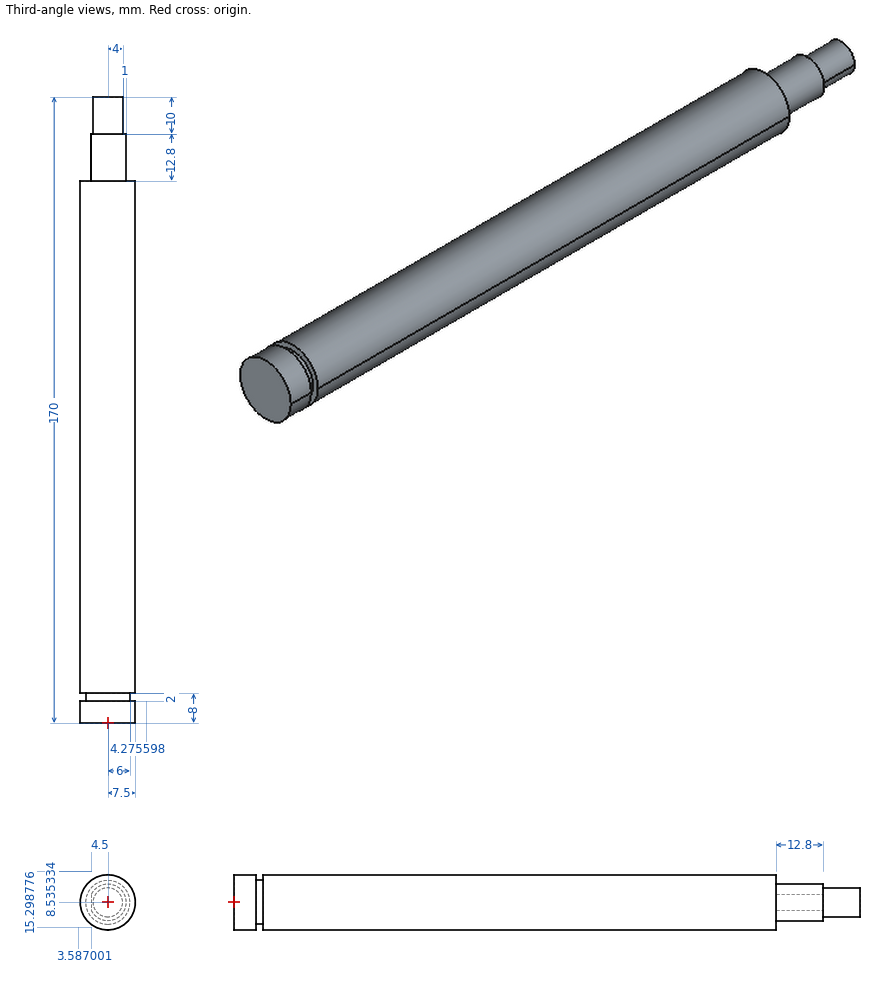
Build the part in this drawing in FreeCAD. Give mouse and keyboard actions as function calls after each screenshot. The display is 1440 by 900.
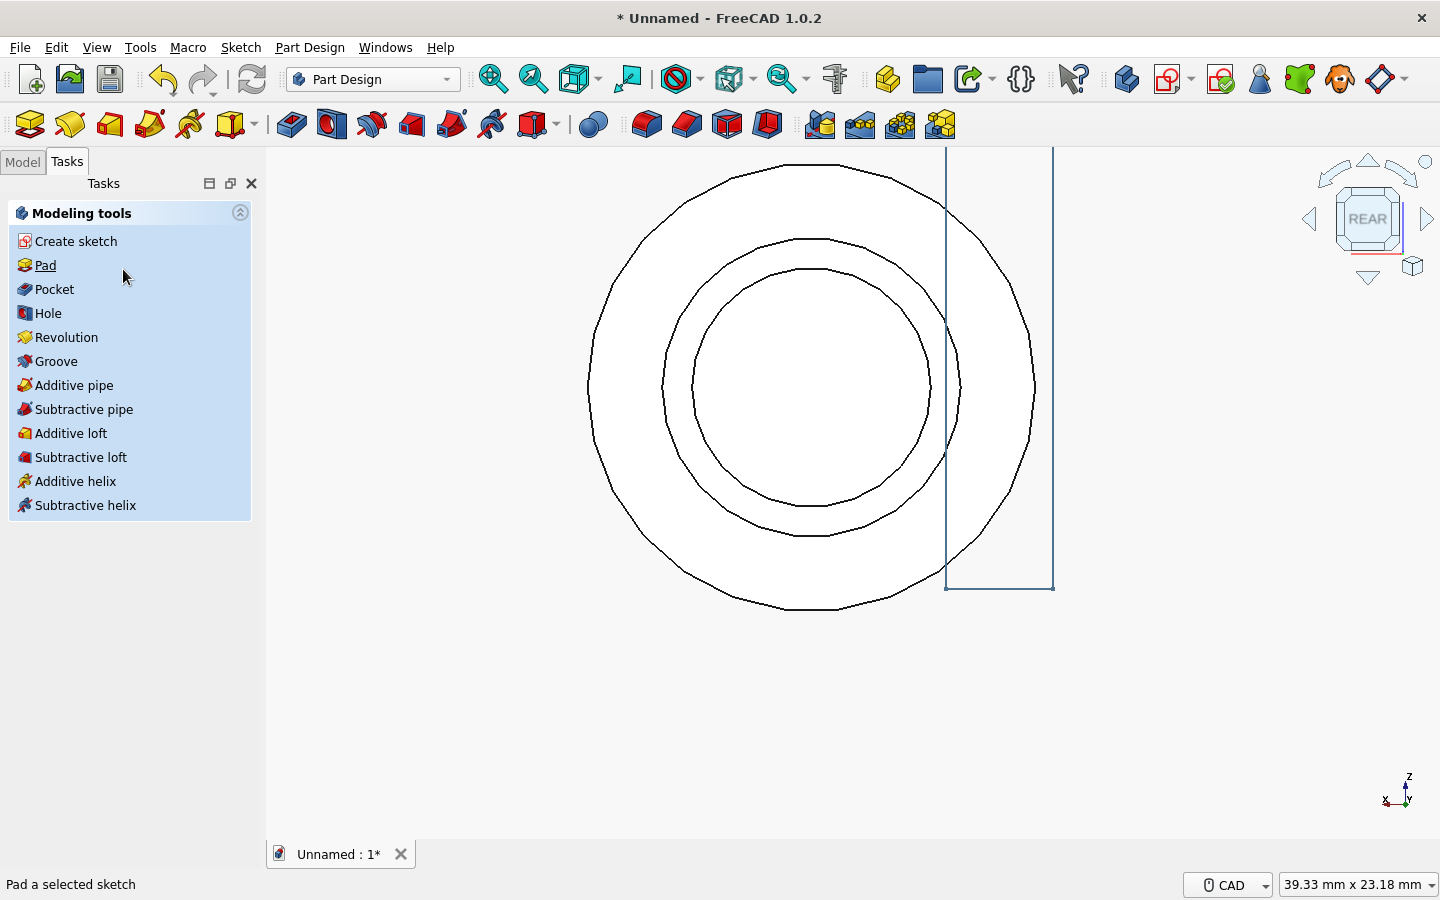
click(292, 124)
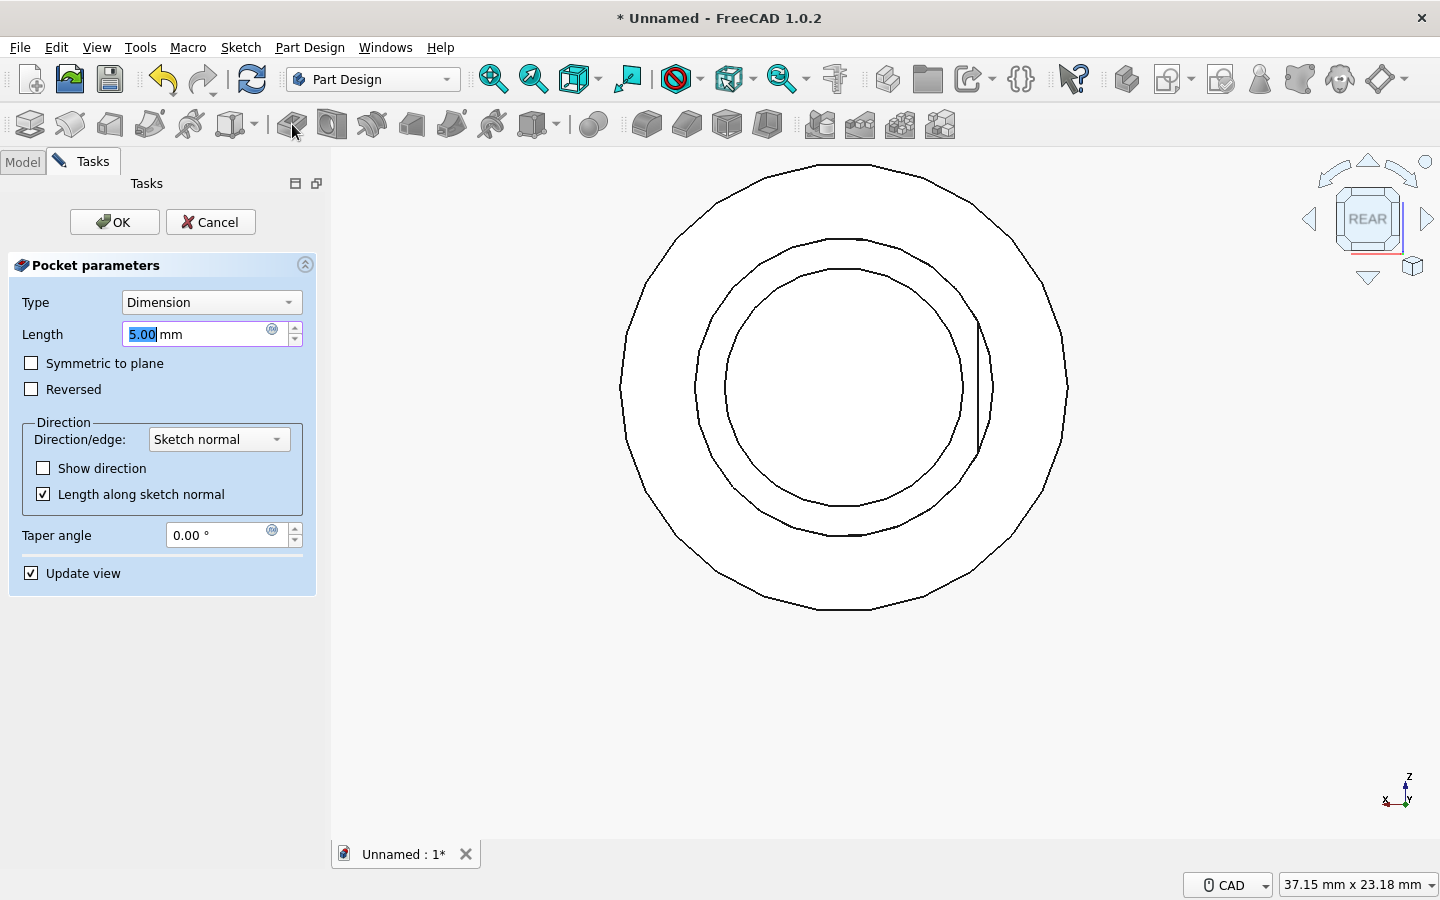
text(12.8)
key(Tab)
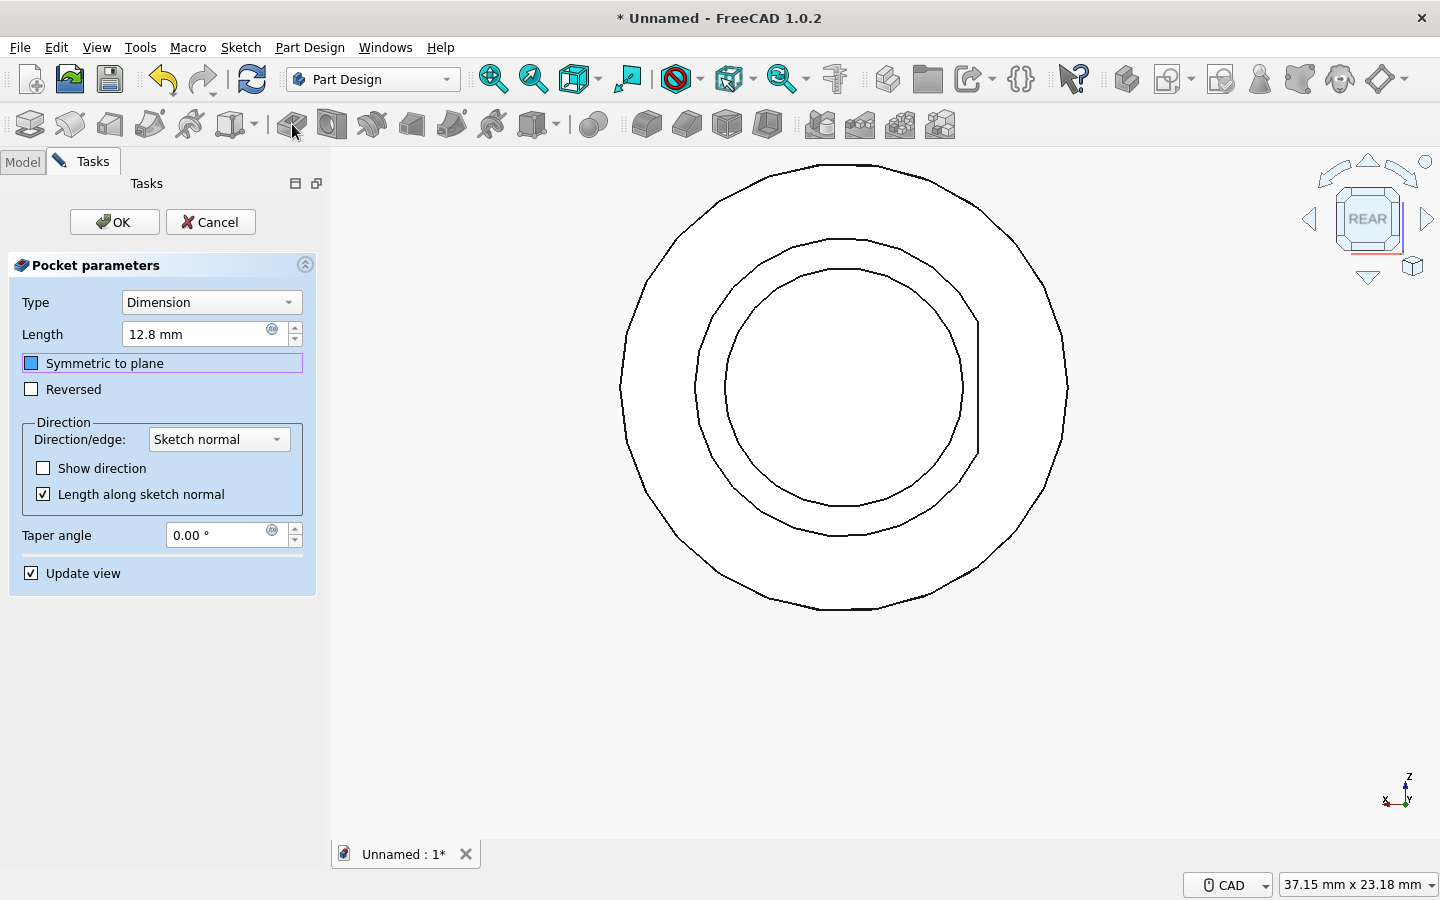
click(115, 222)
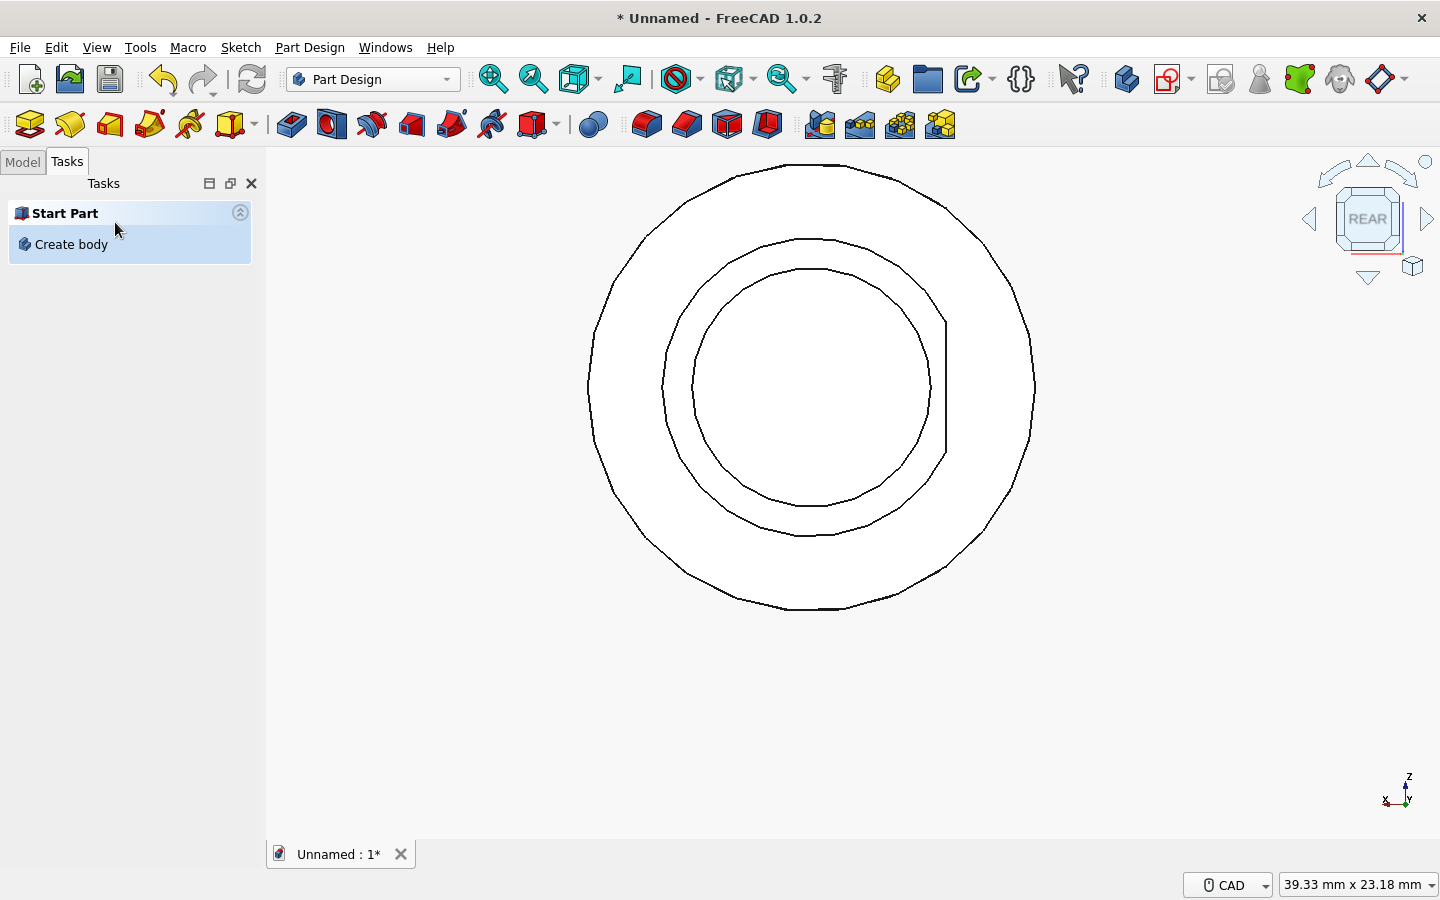
click(1168, 80)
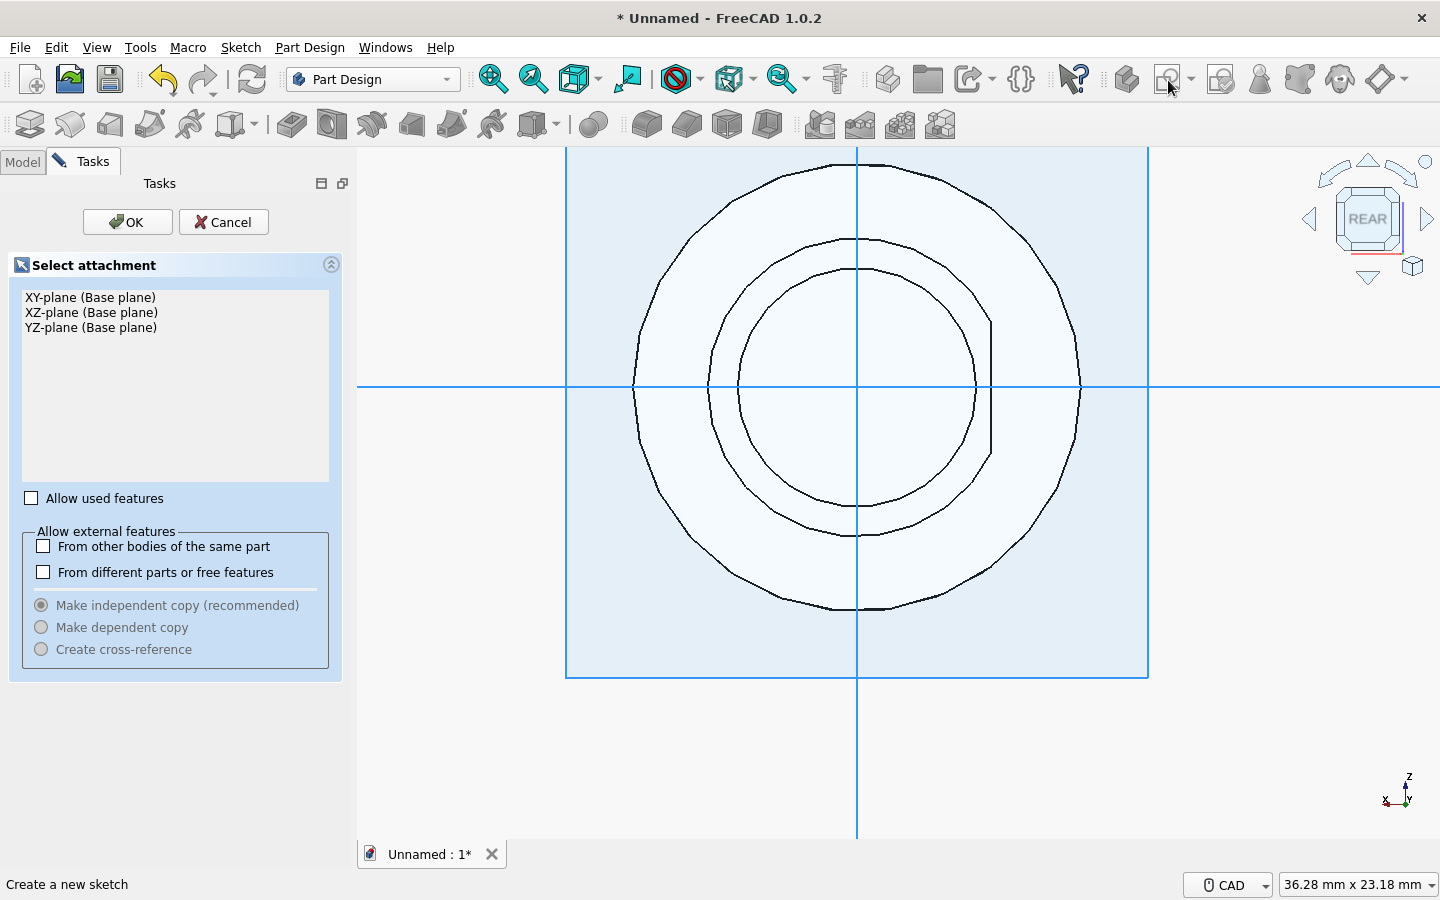
click(82, 298)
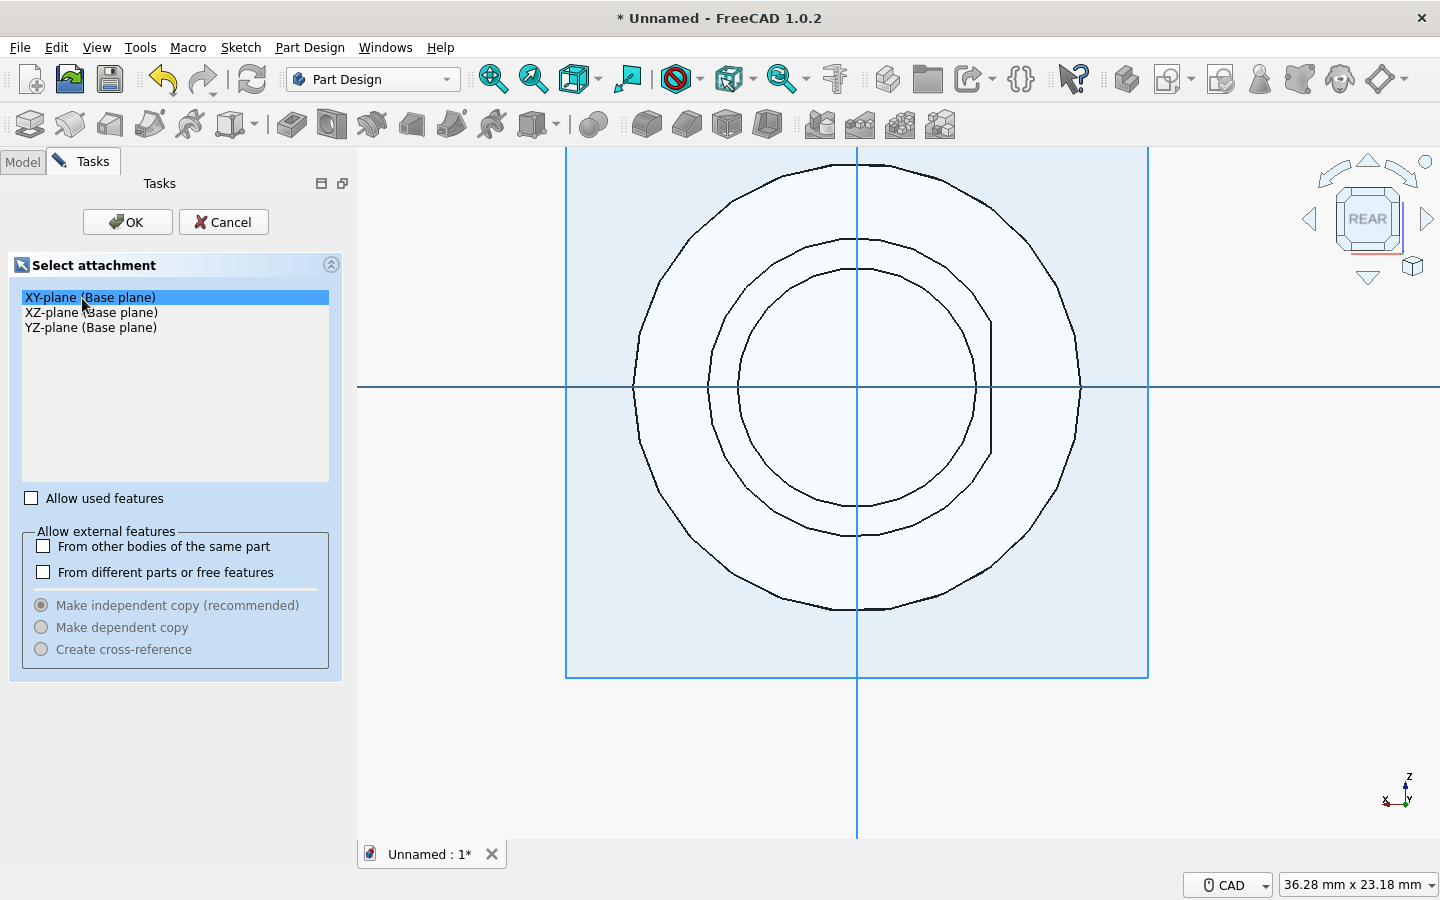
click(128, 222)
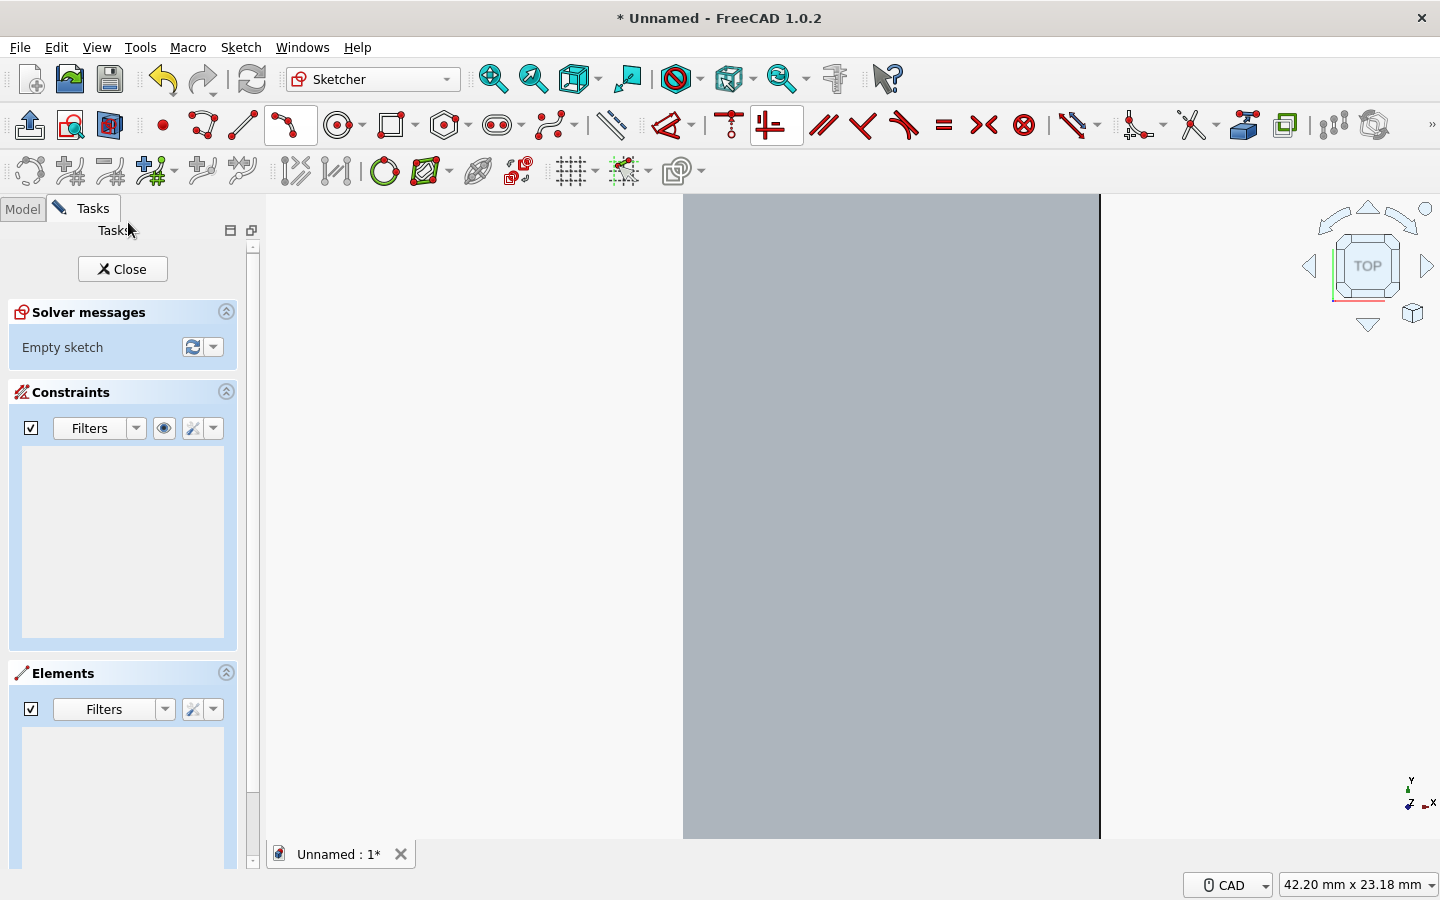
click(110, 126)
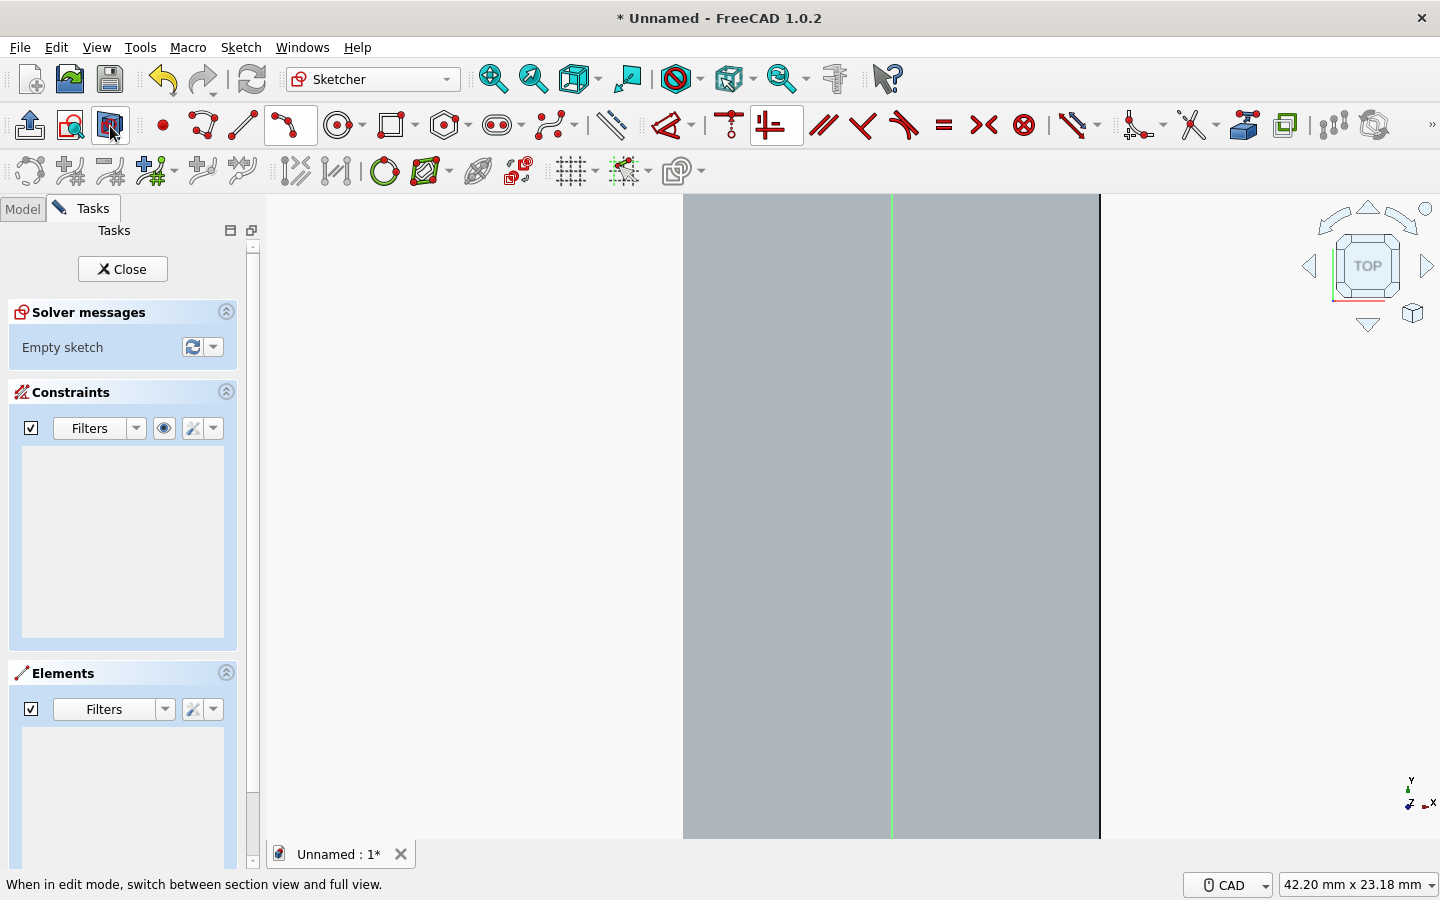
scroll(784, 516, down, 5)